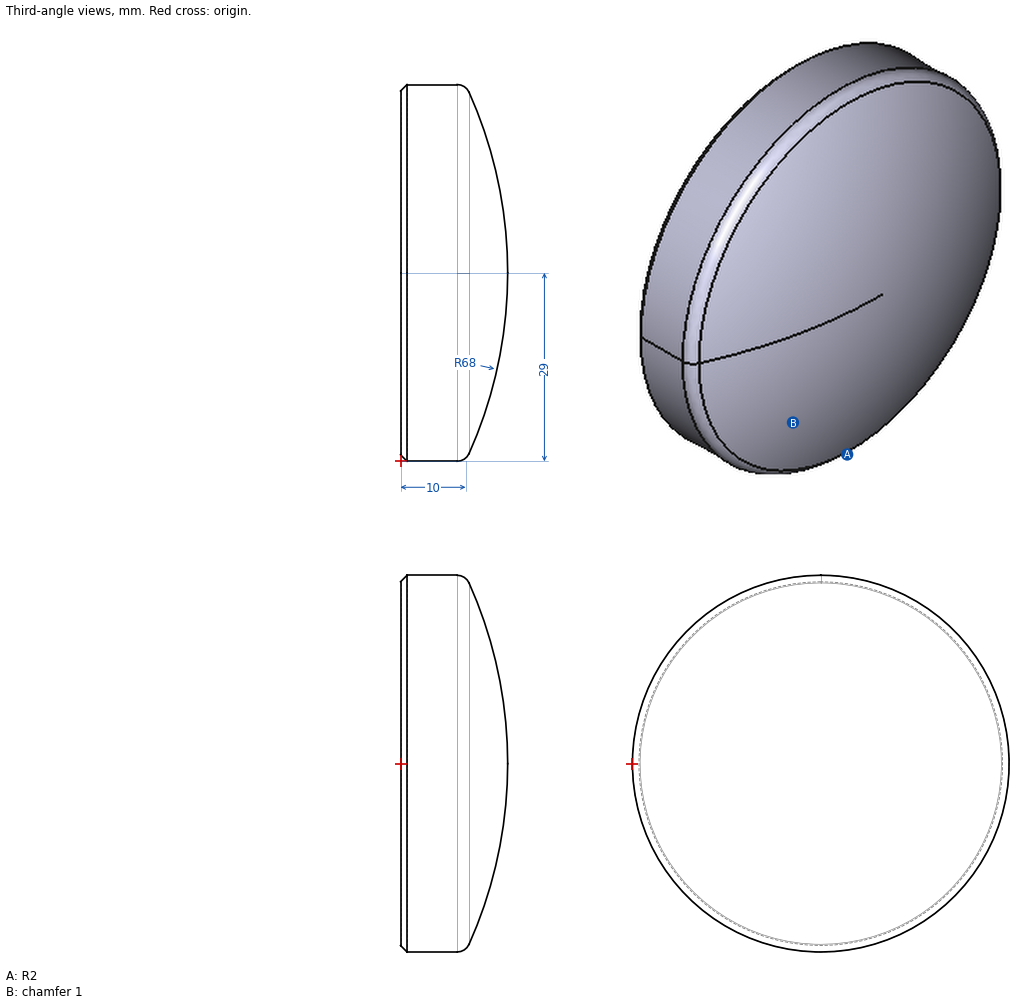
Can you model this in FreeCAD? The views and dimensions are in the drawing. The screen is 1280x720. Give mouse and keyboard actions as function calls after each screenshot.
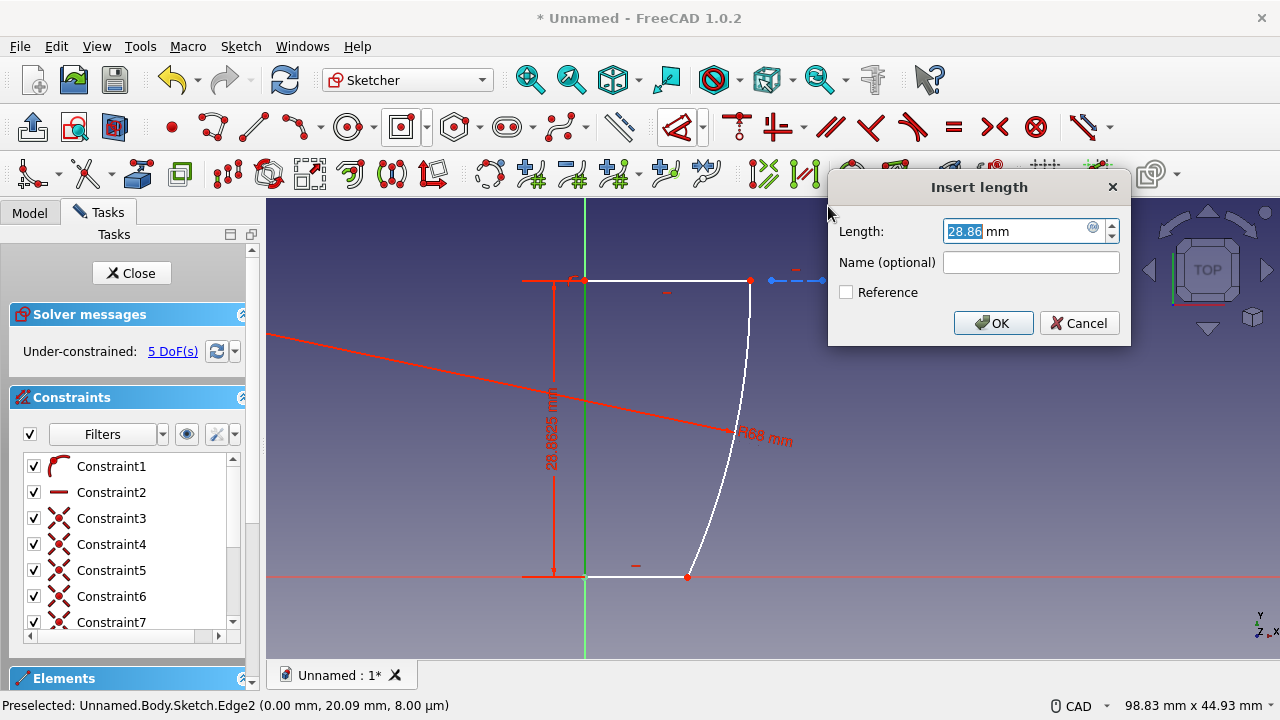
text(29)
key(Return)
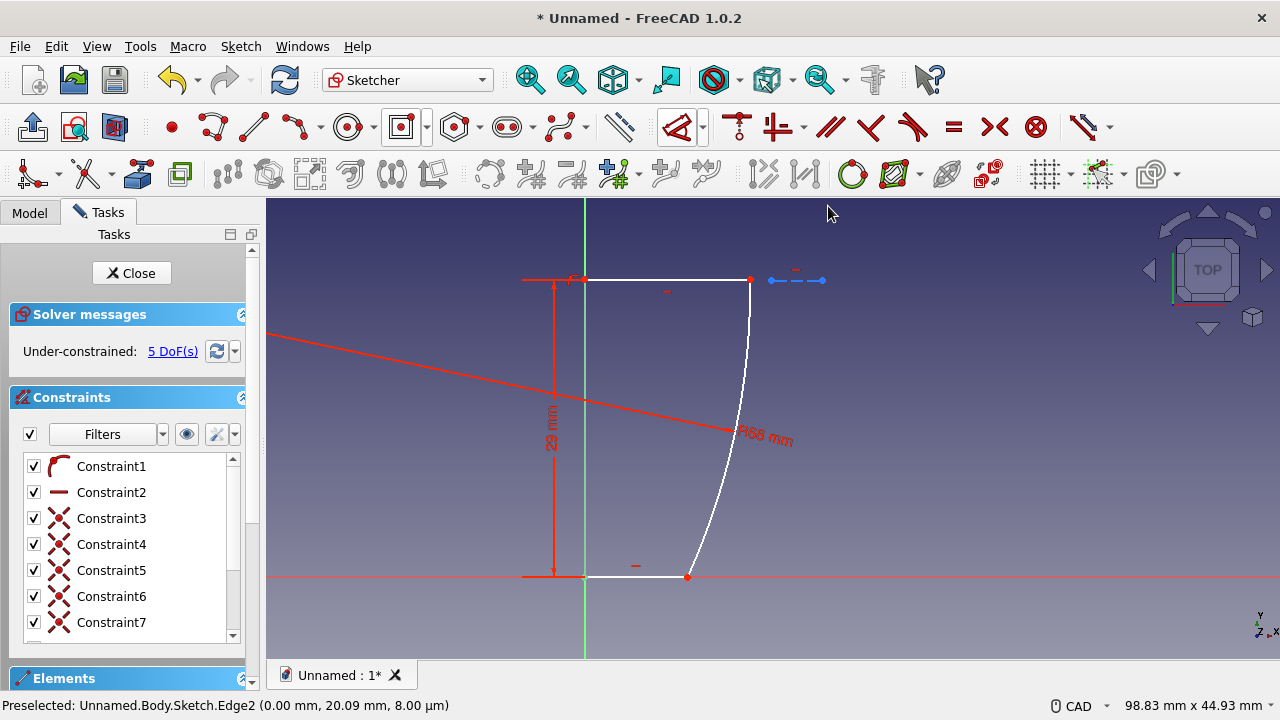
click(616, 577)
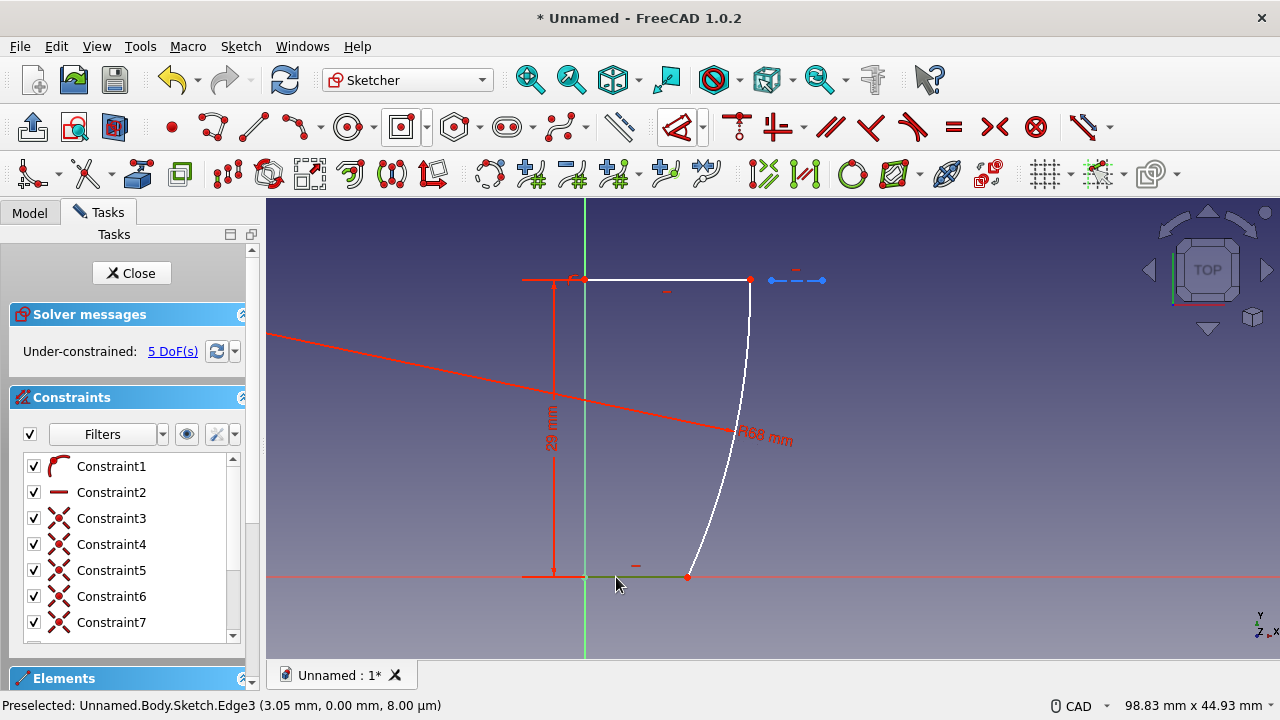
click(702, 128)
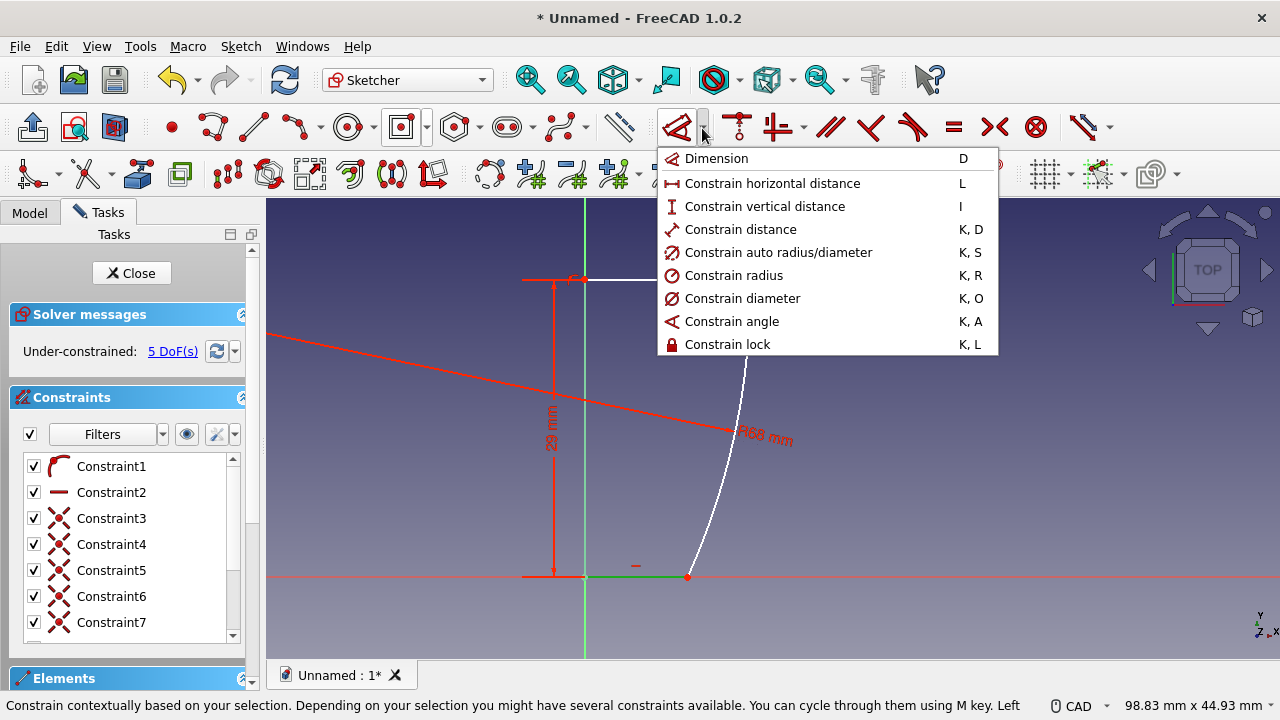
click(828, 184)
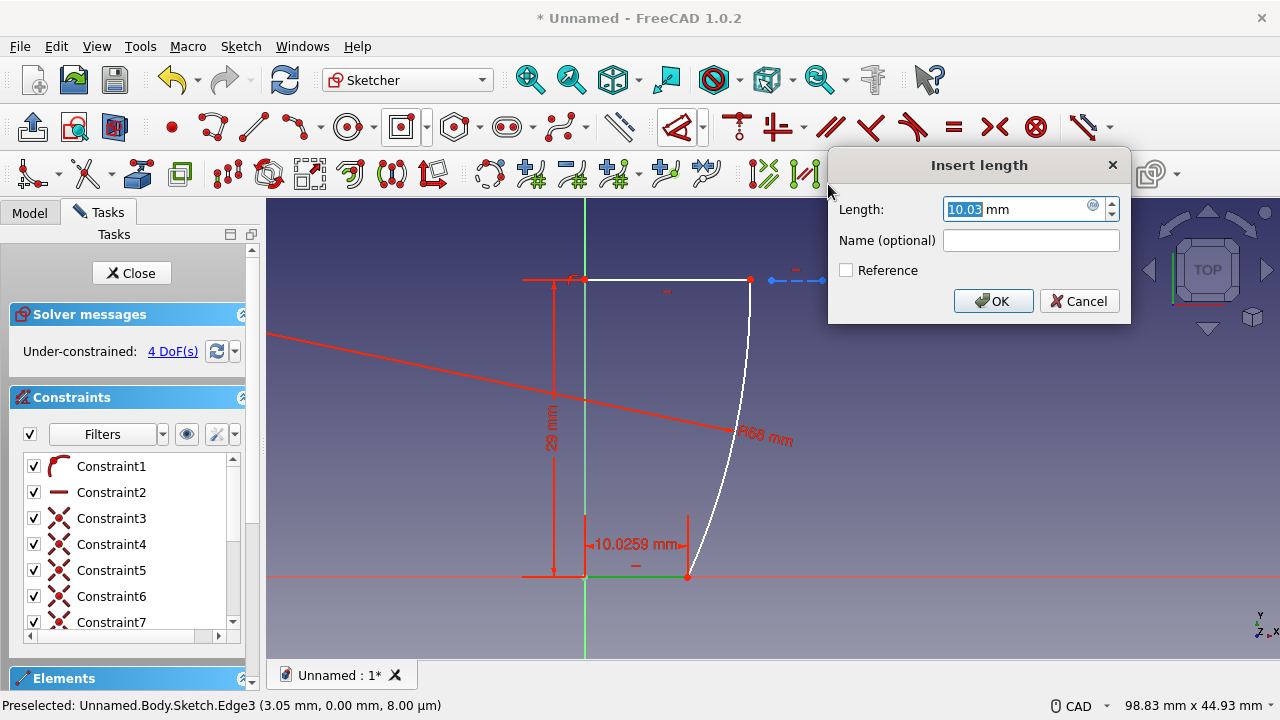
text(10)
key(Return)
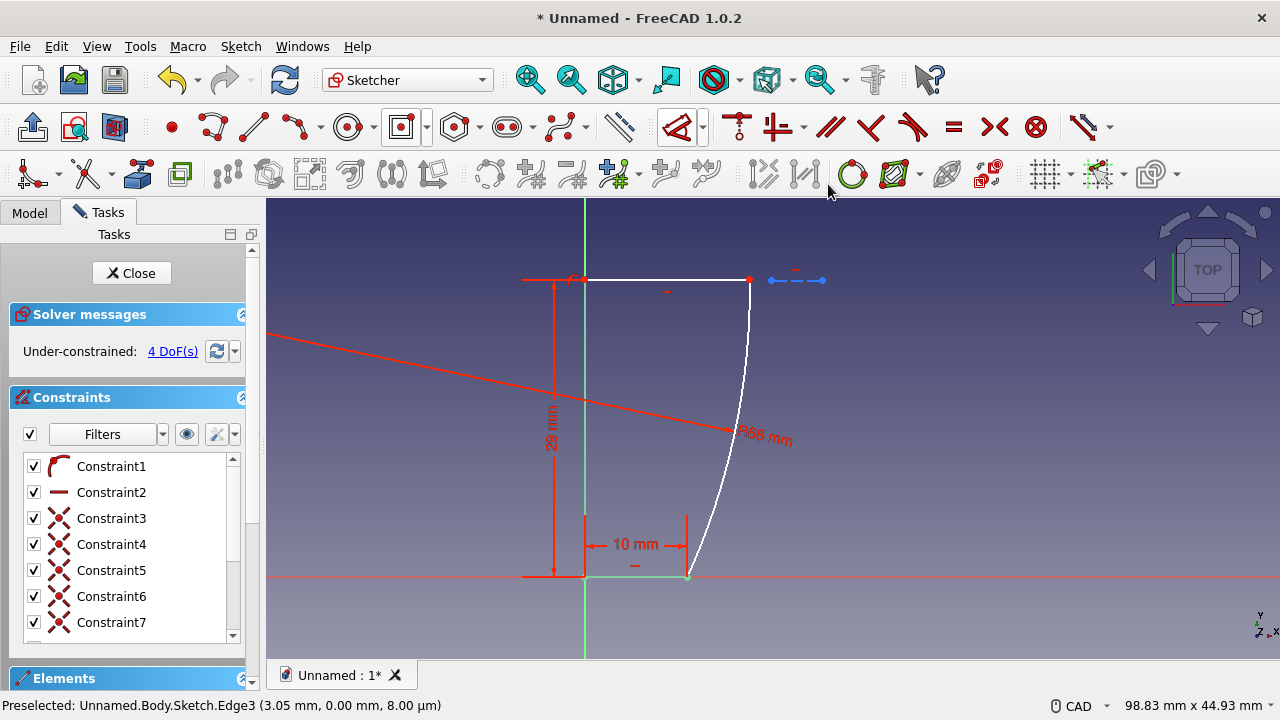
click(771, 281)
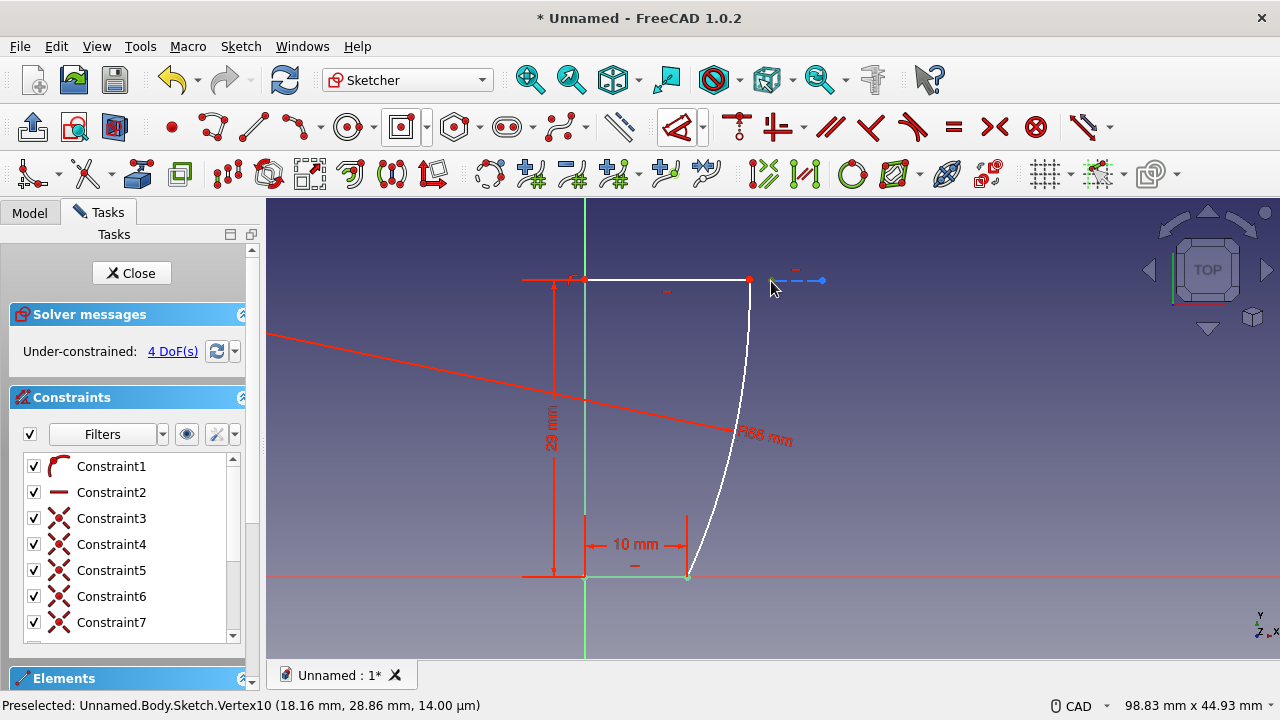
click(702, 128)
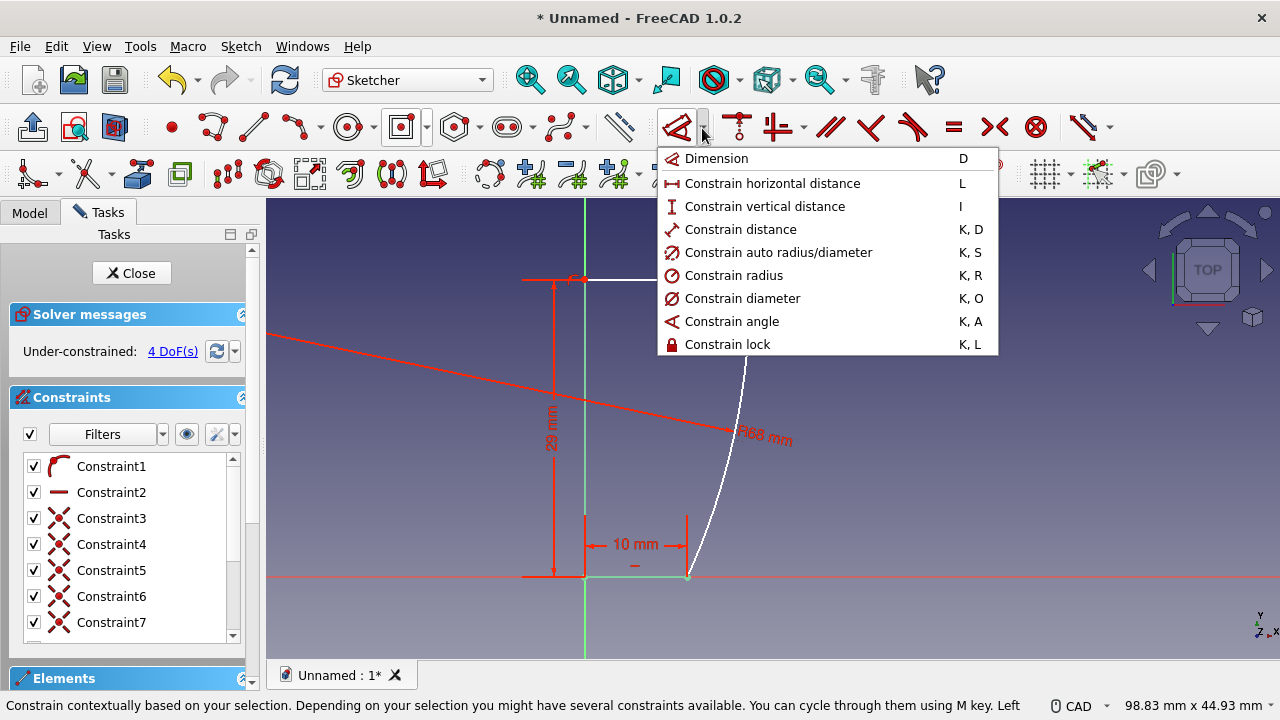
click(828, 206)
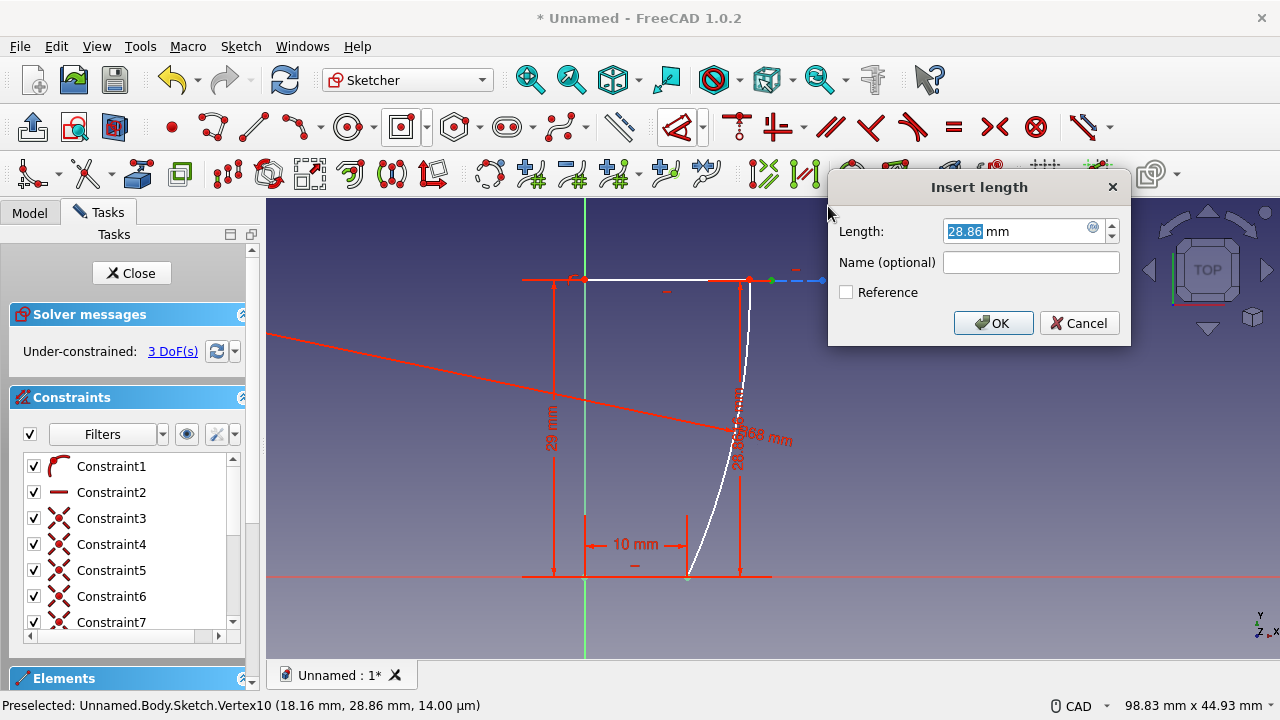
text(29)
key(Return)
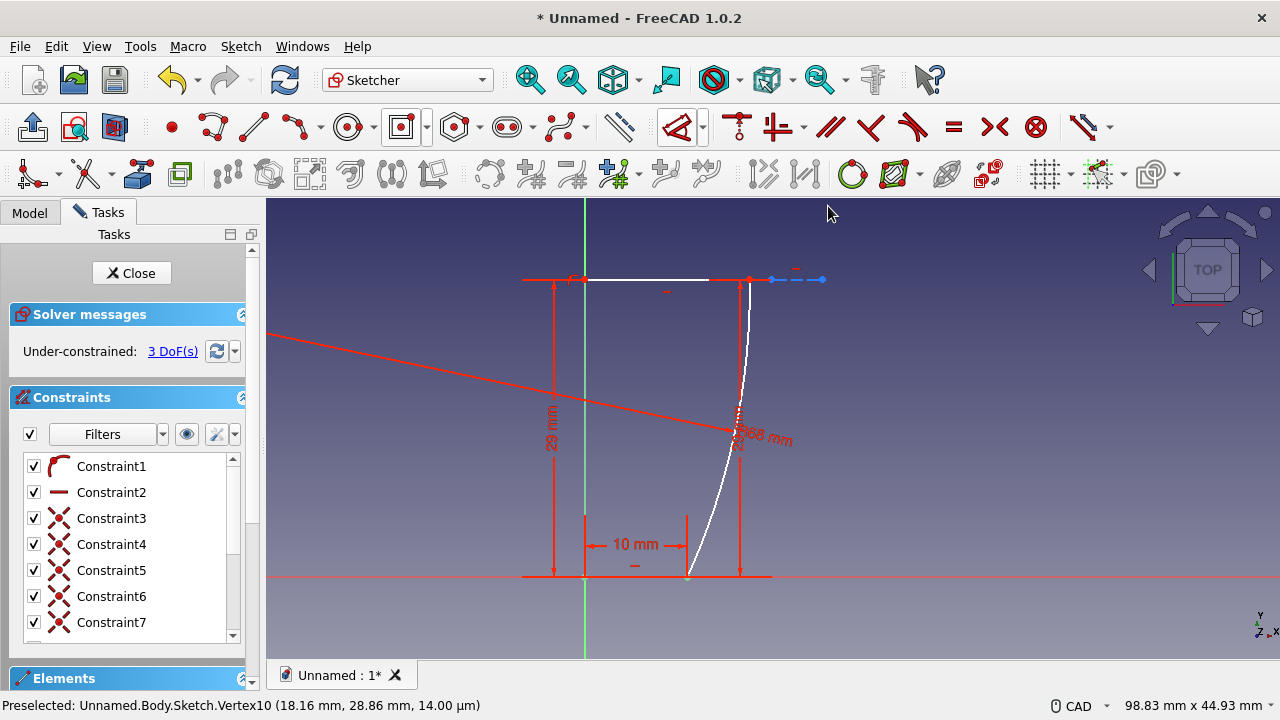
scroll(1115, 429, down, 2)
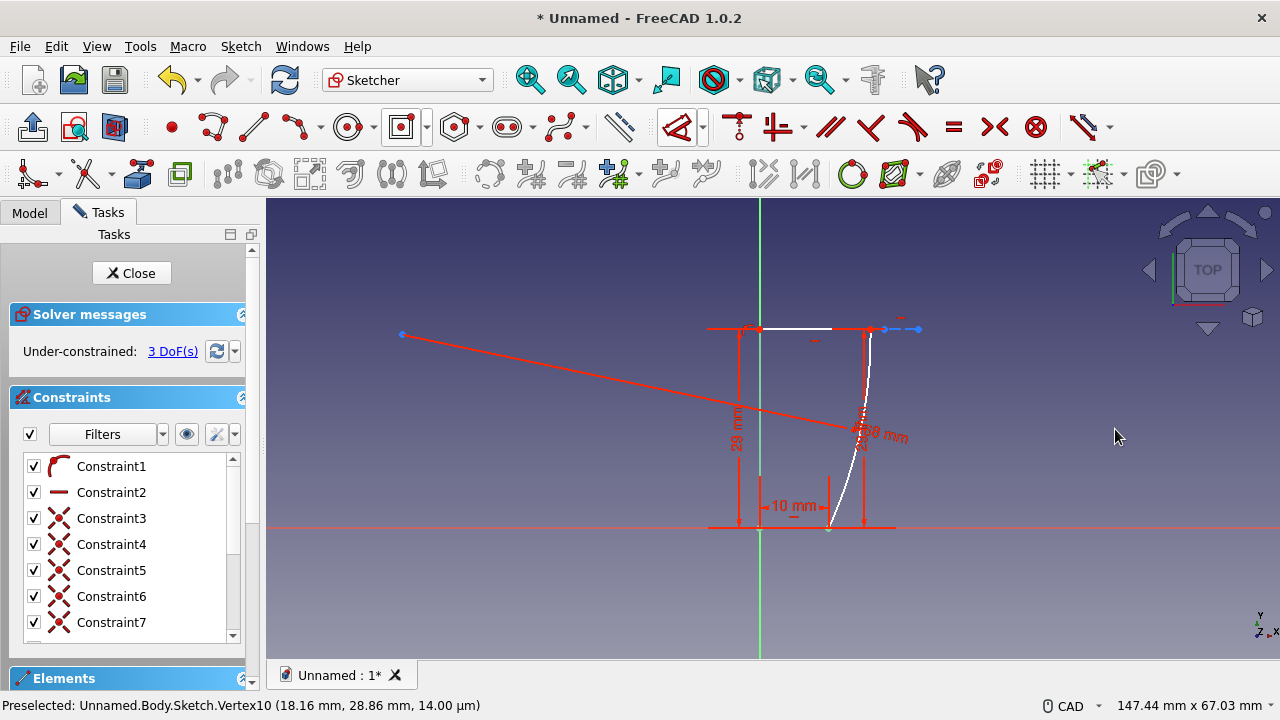
click(403, 335)